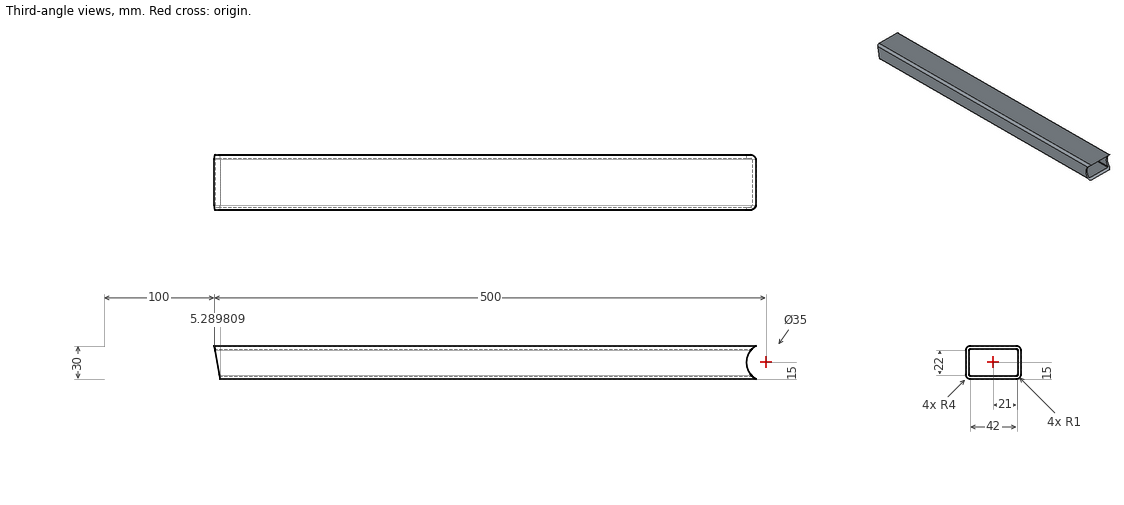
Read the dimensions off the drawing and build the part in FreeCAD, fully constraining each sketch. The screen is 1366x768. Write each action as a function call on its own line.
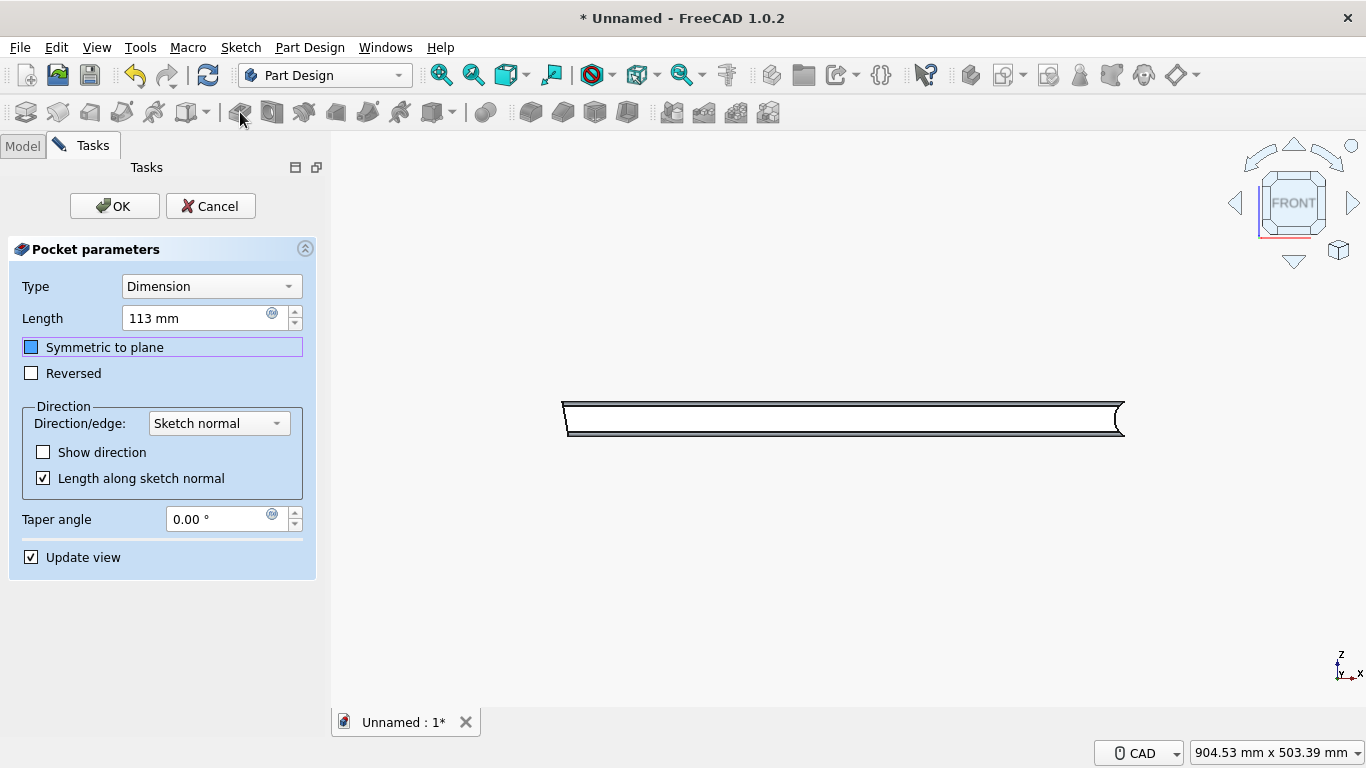
click(115, 206)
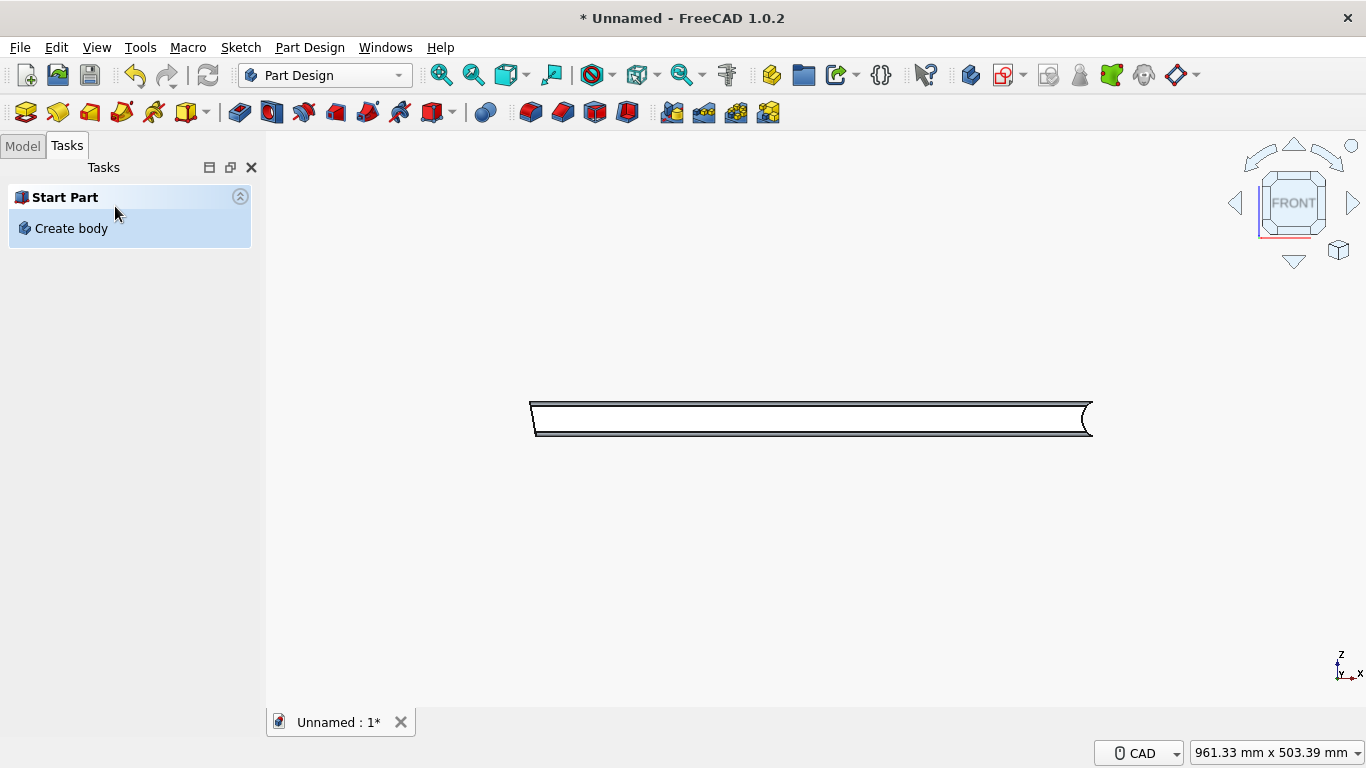
key(0)